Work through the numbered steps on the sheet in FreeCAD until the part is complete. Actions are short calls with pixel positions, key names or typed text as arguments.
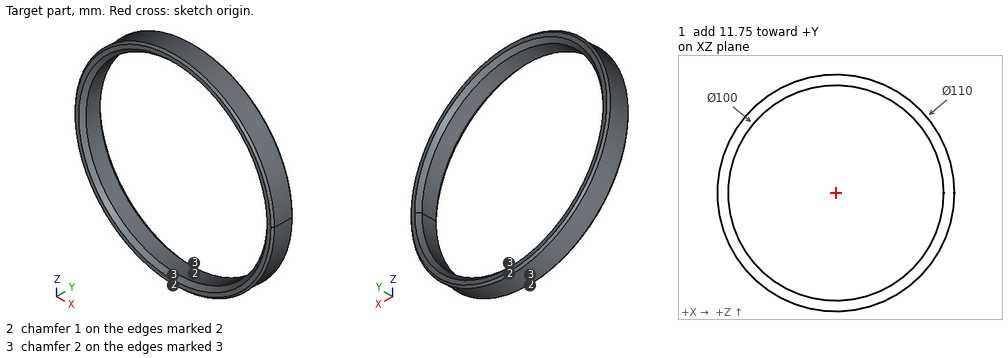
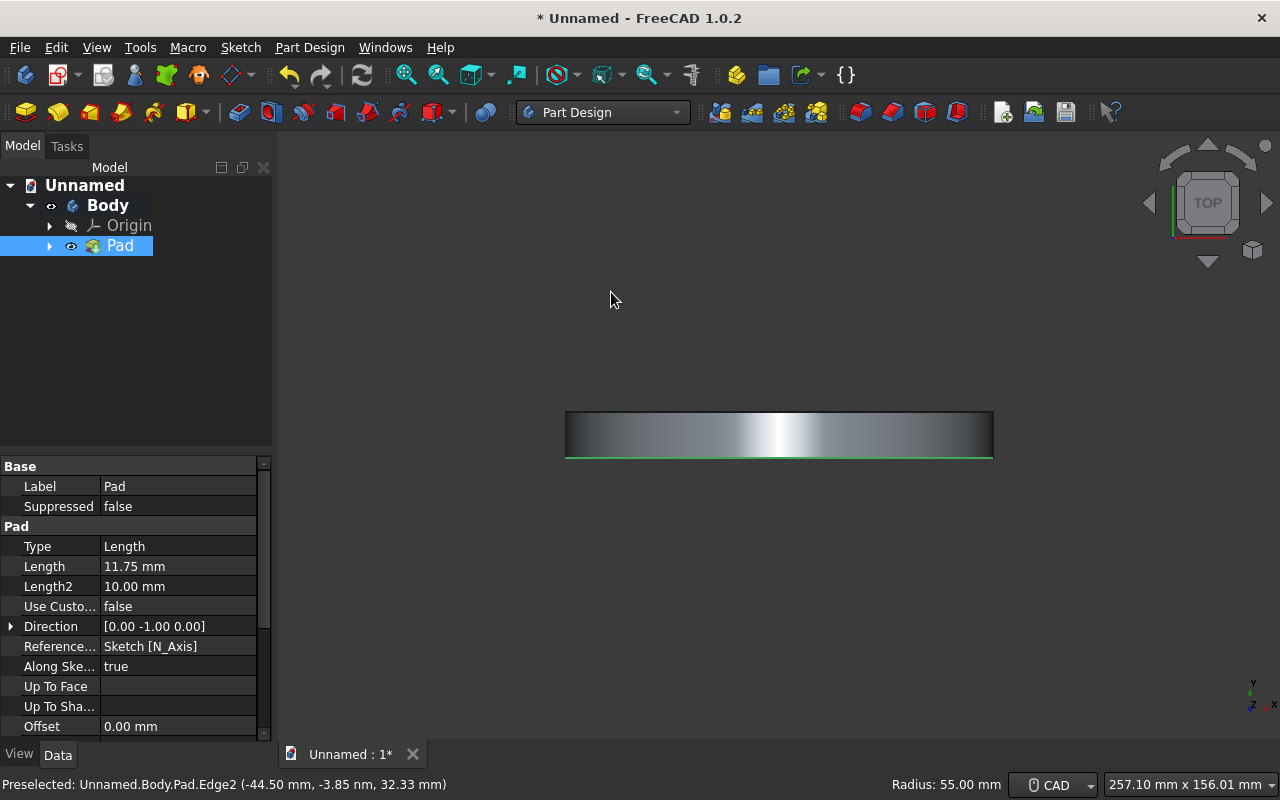
click(606, 411, ctrl)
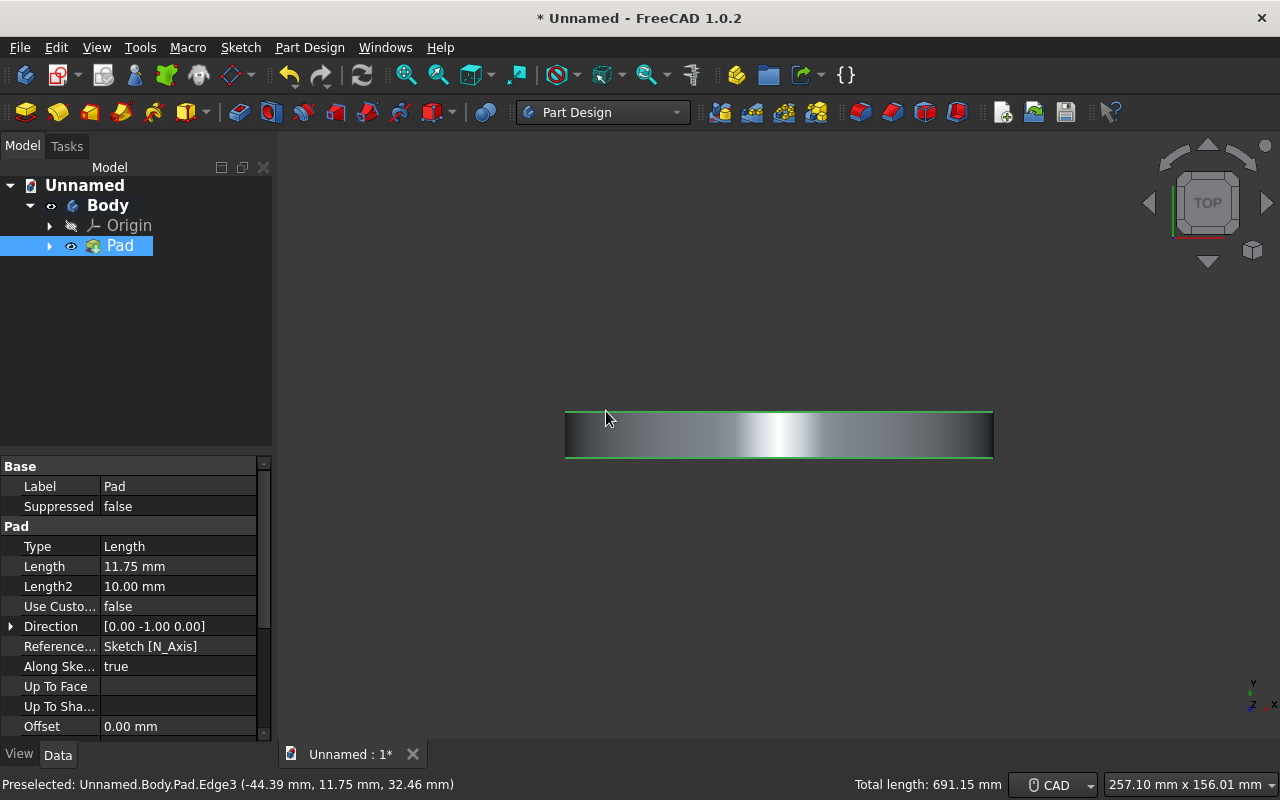
click(894, 112)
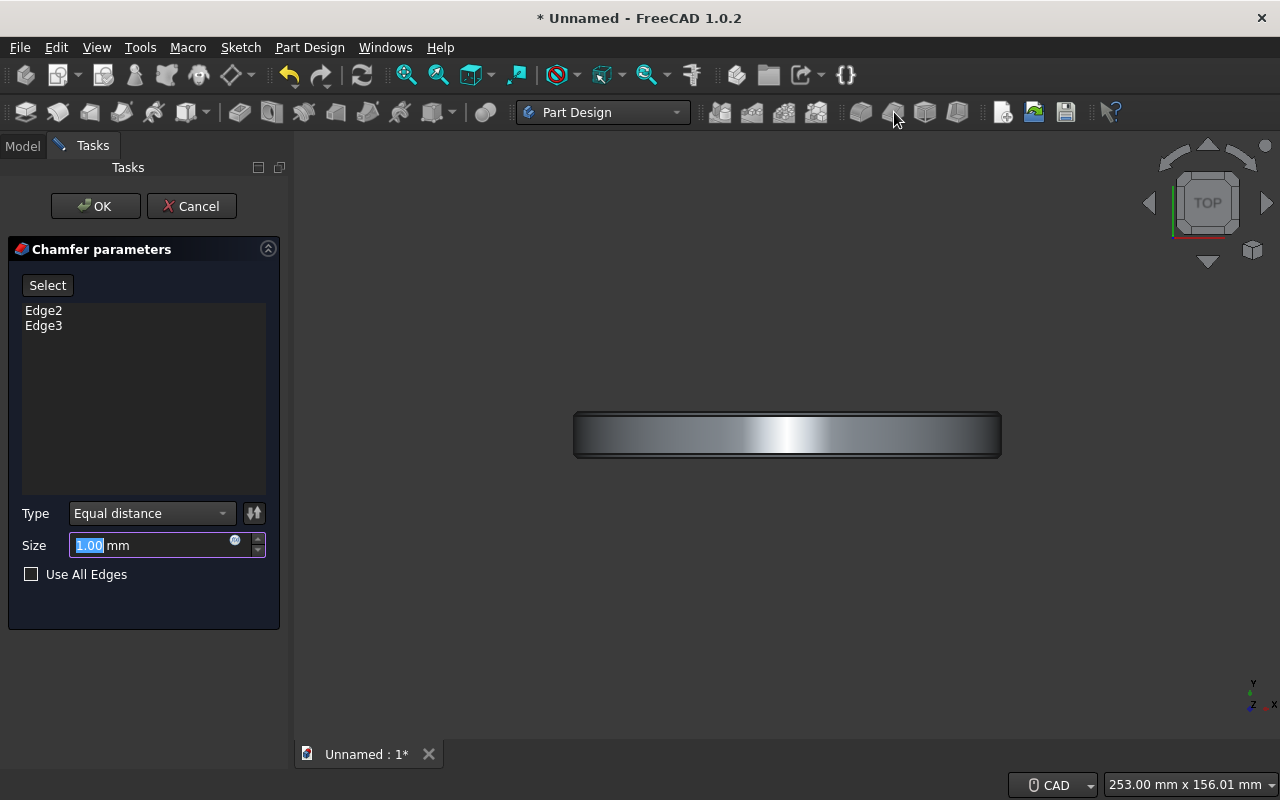
text(1)
key(Tab)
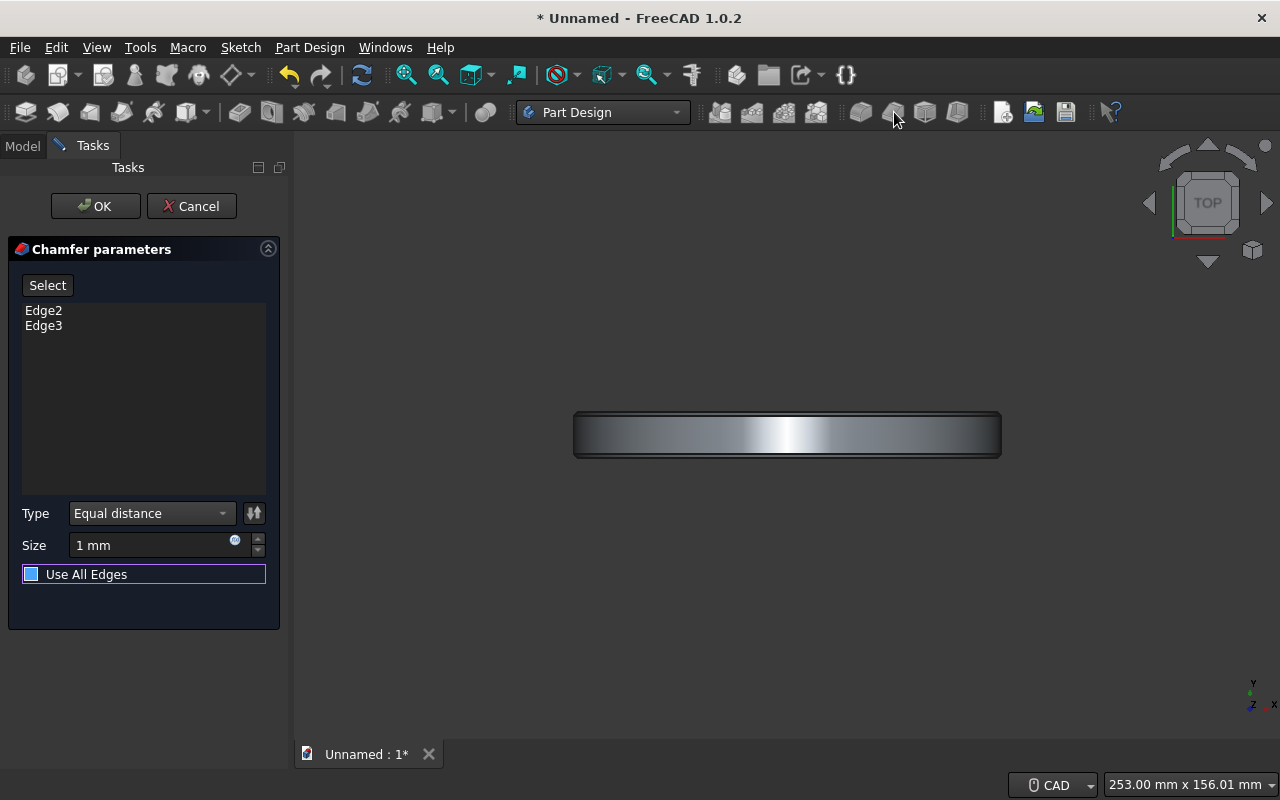
click(96, 206)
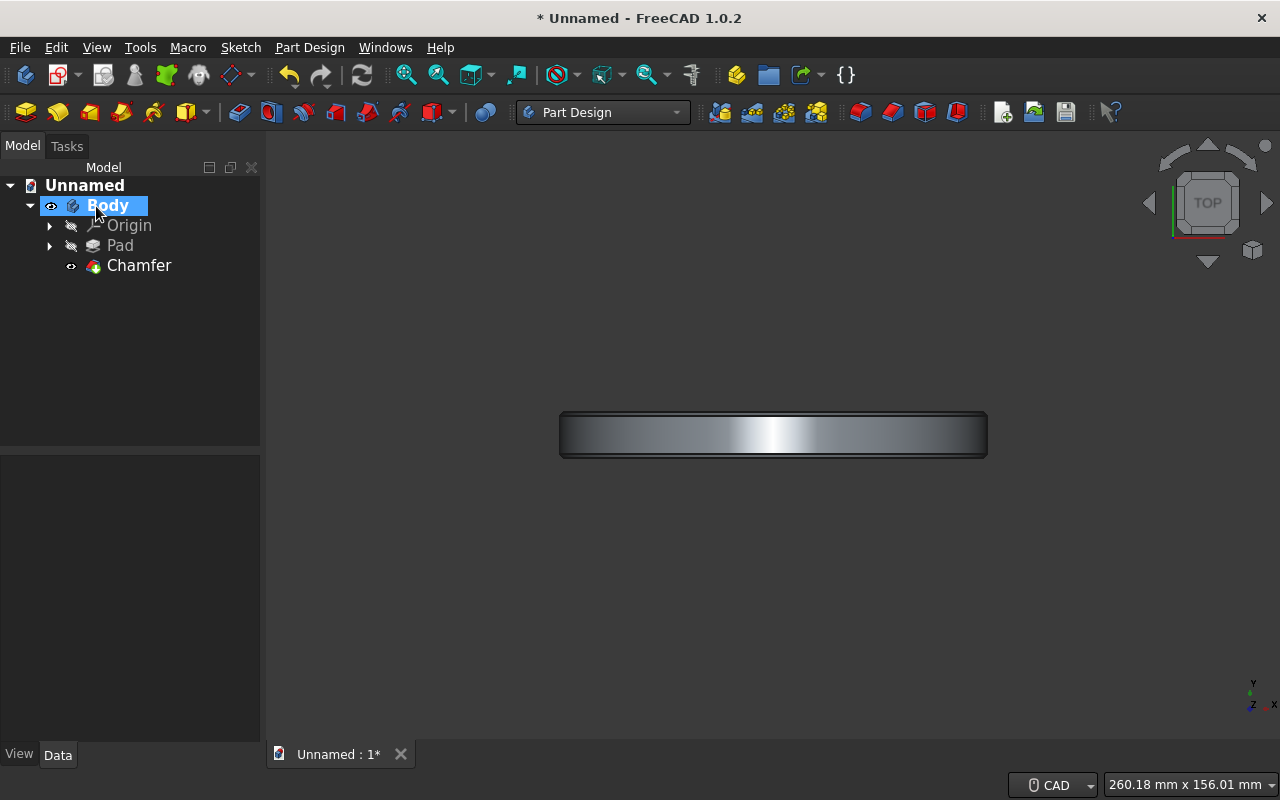
click(408, 76)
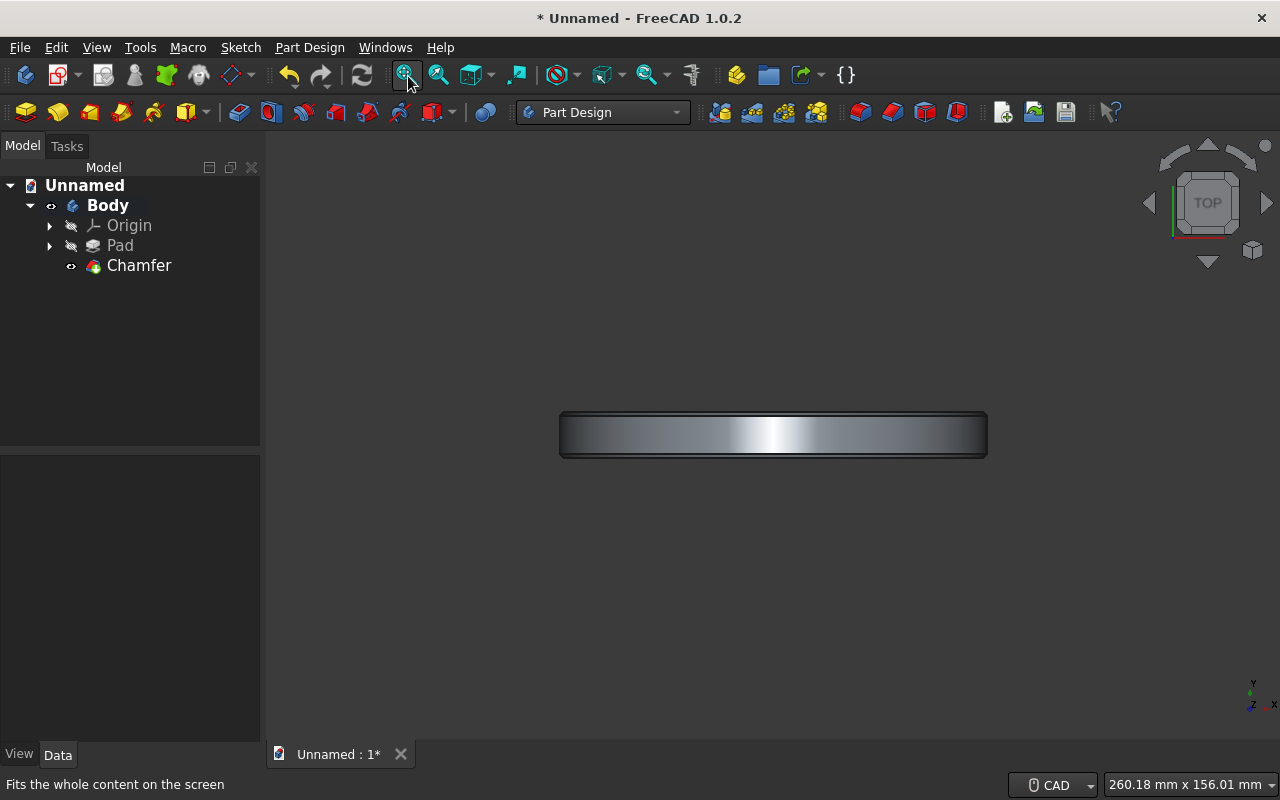
key(0)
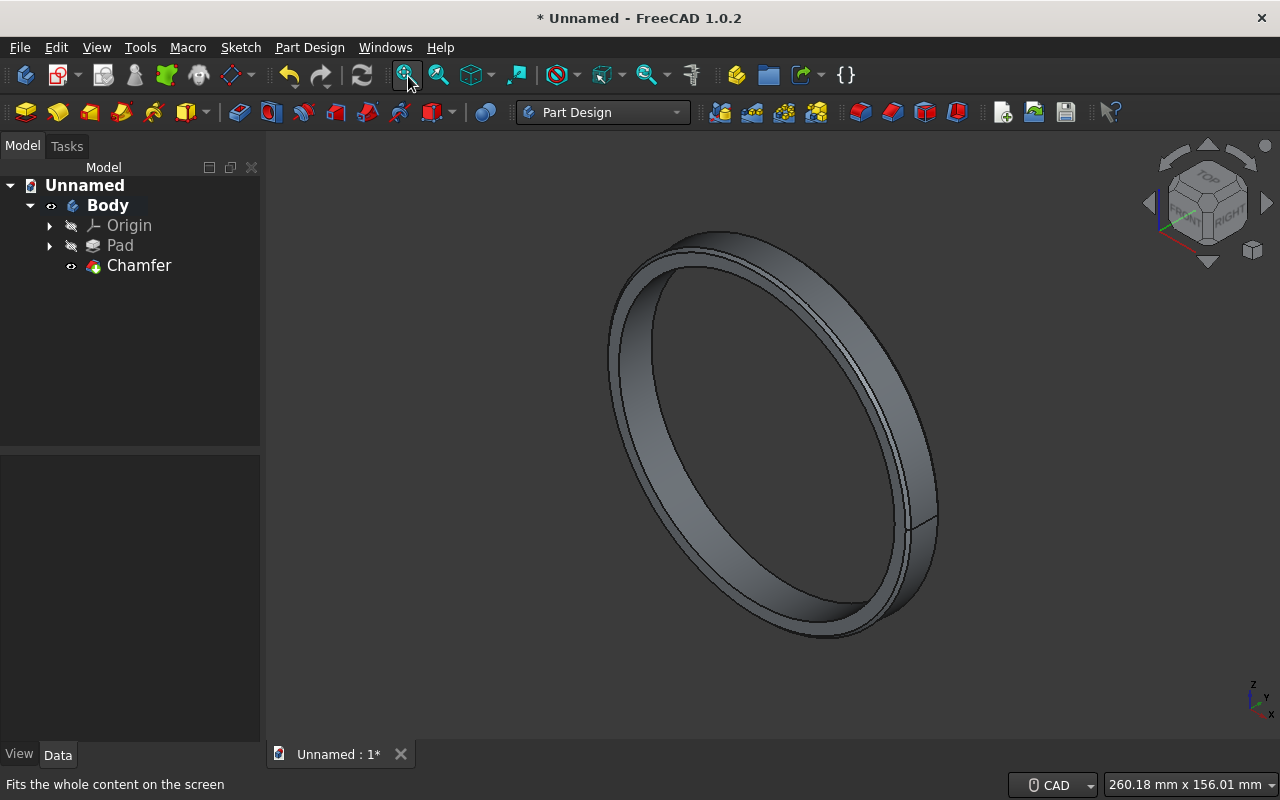
click(619, 364)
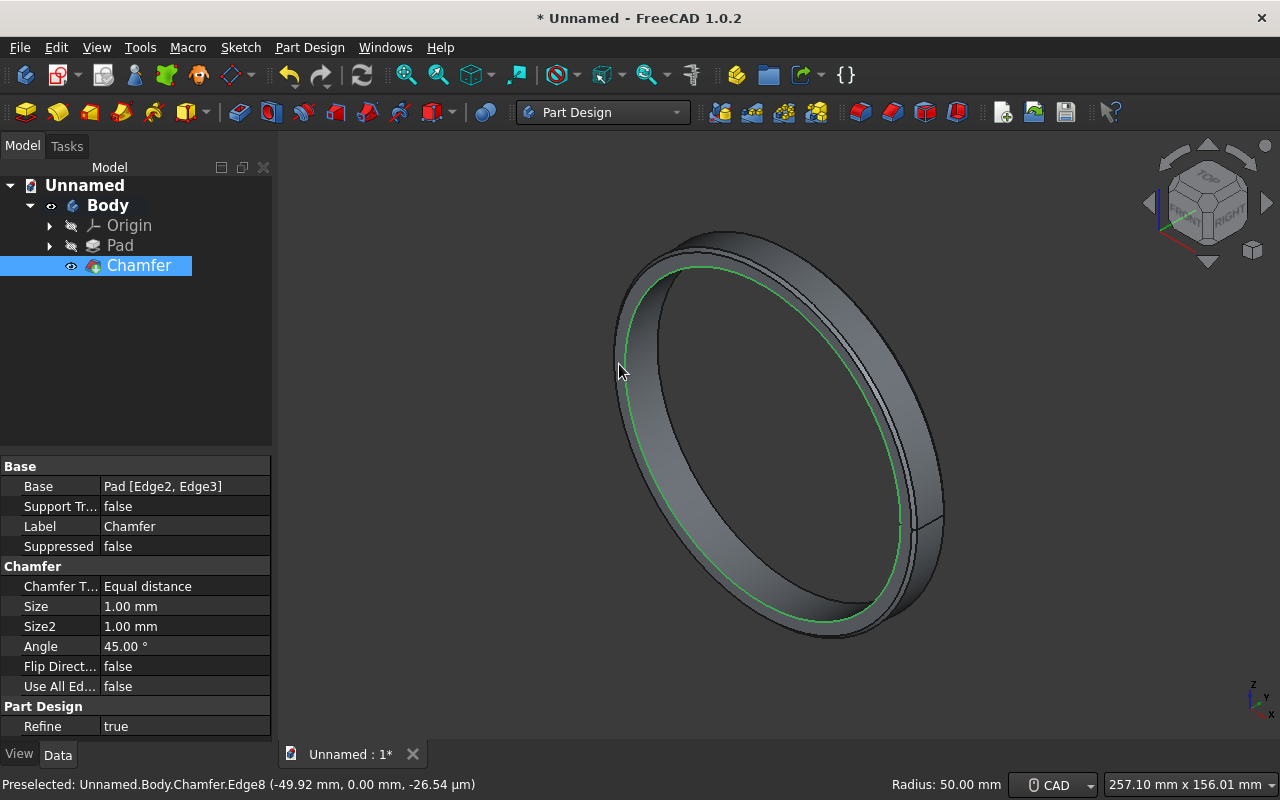
key(2)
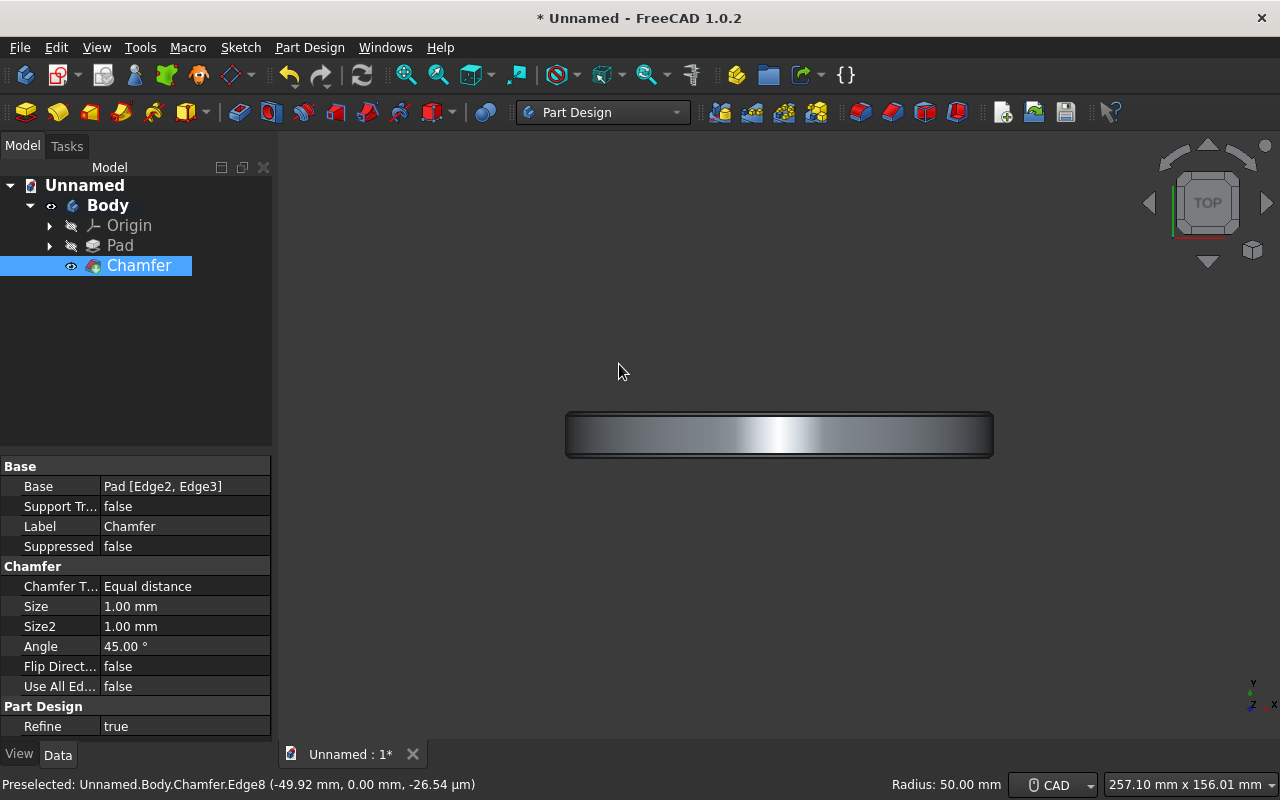
key(v)
key(f)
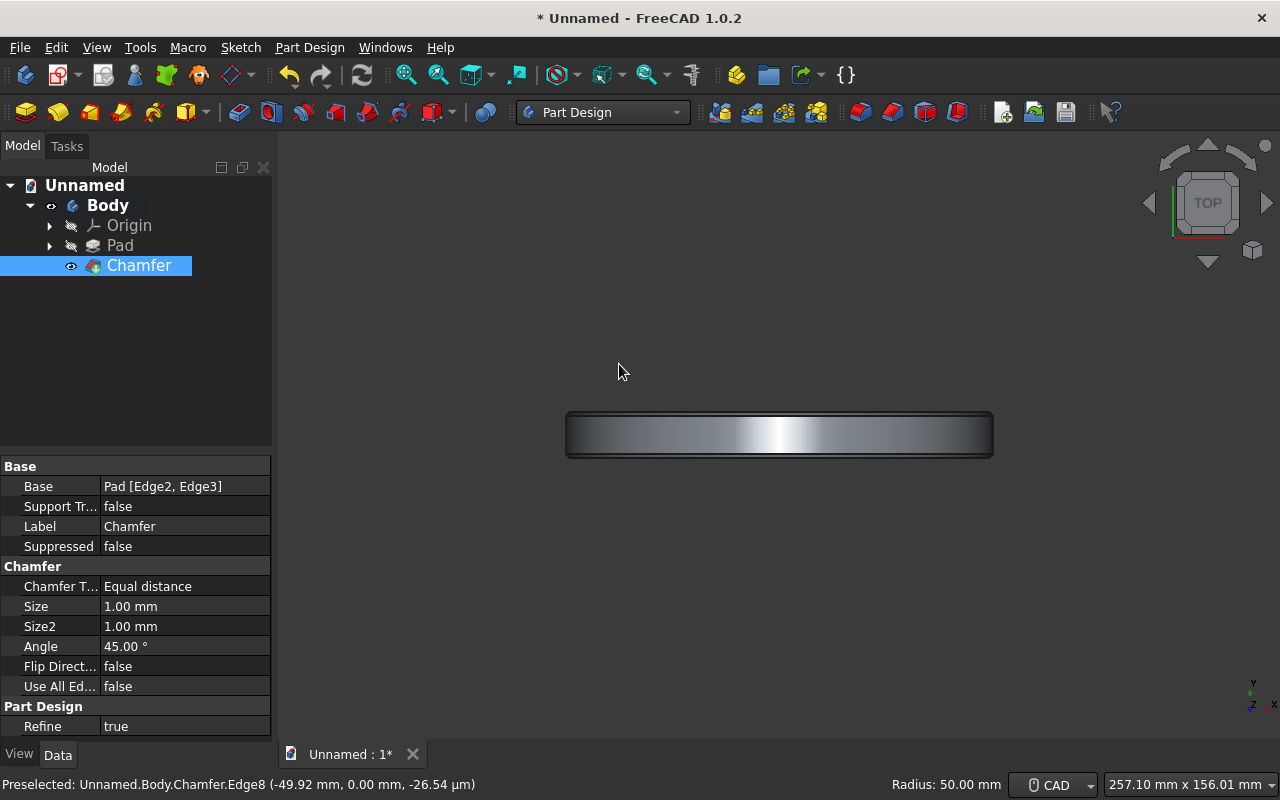
key(1)